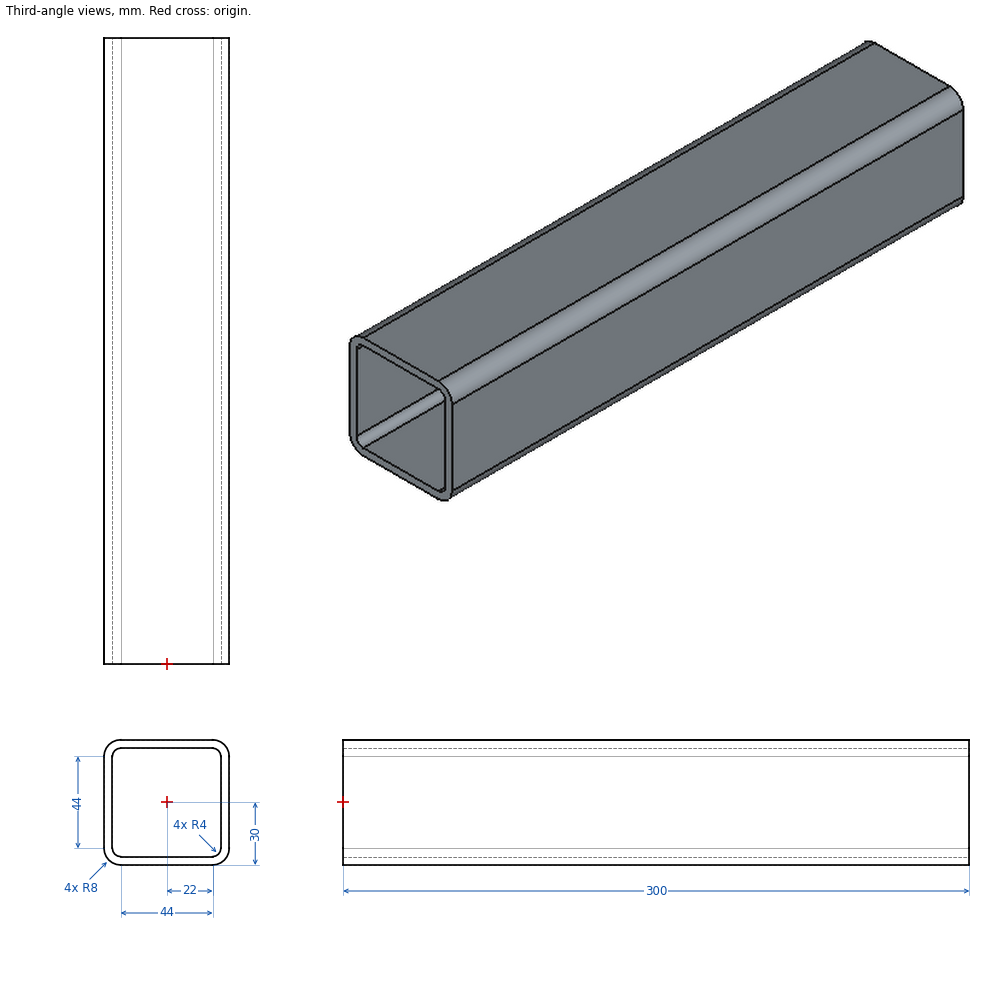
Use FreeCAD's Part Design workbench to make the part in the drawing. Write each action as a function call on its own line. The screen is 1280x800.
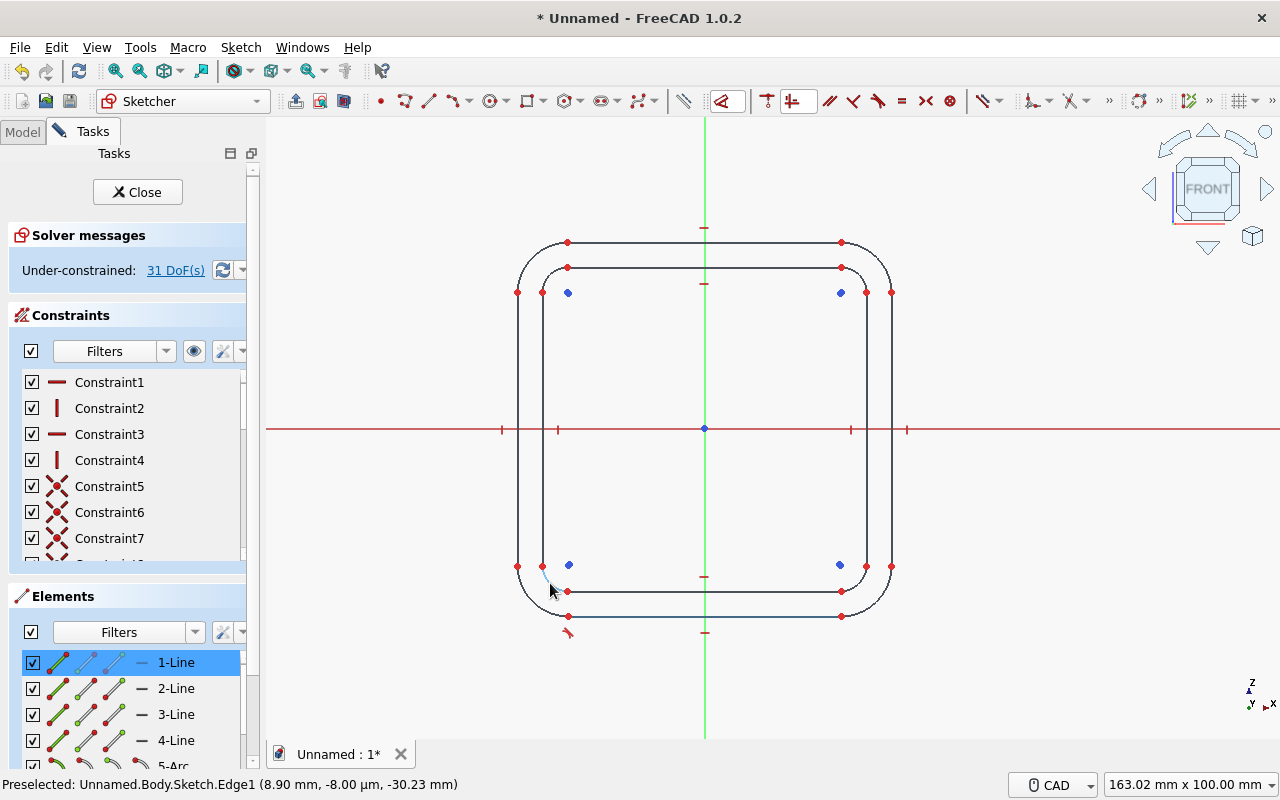
click(864, 611)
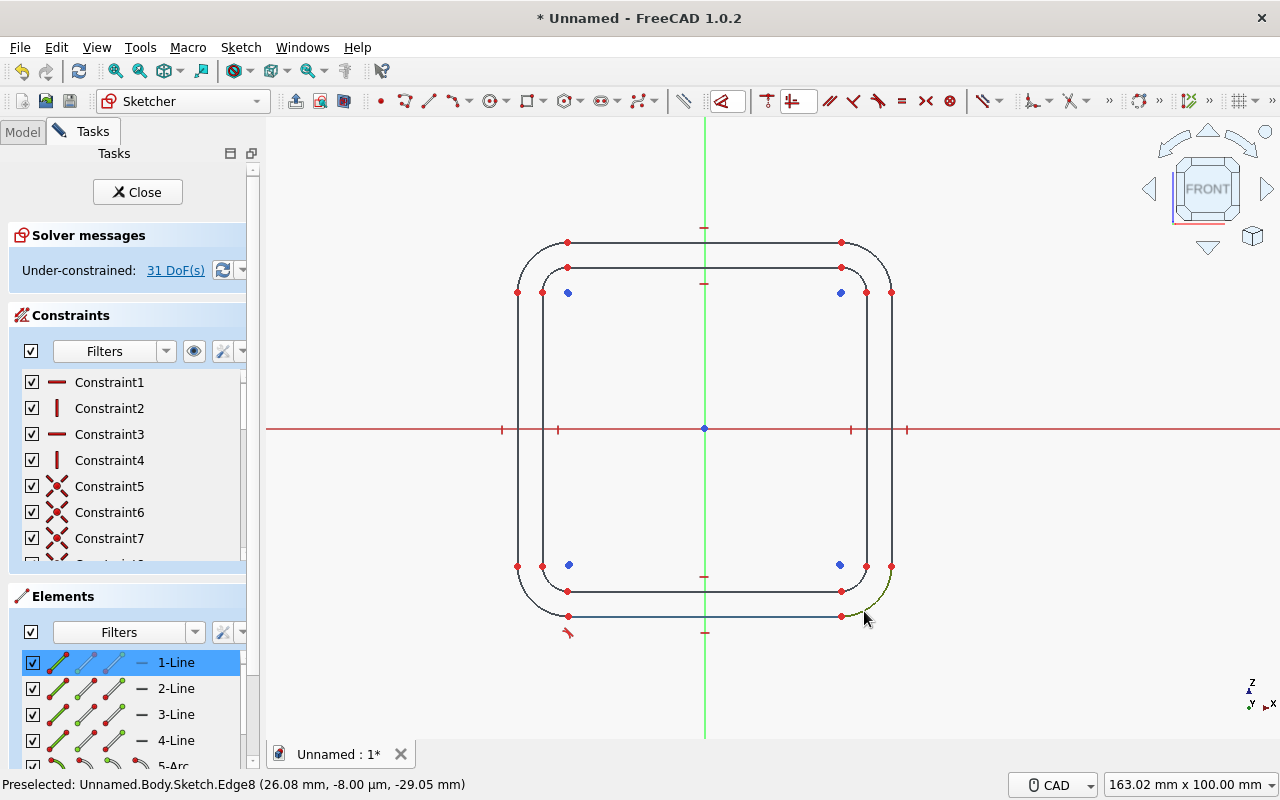
key(t)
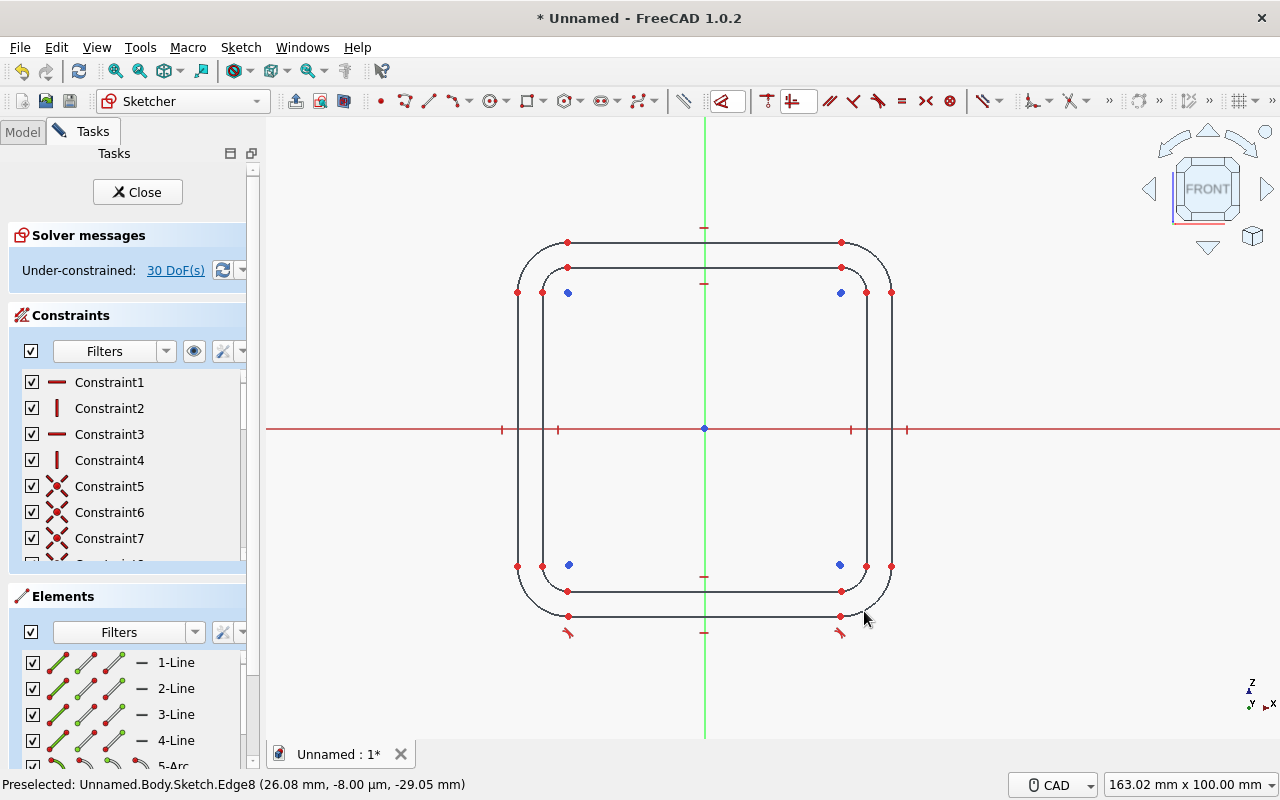
click(518, 484)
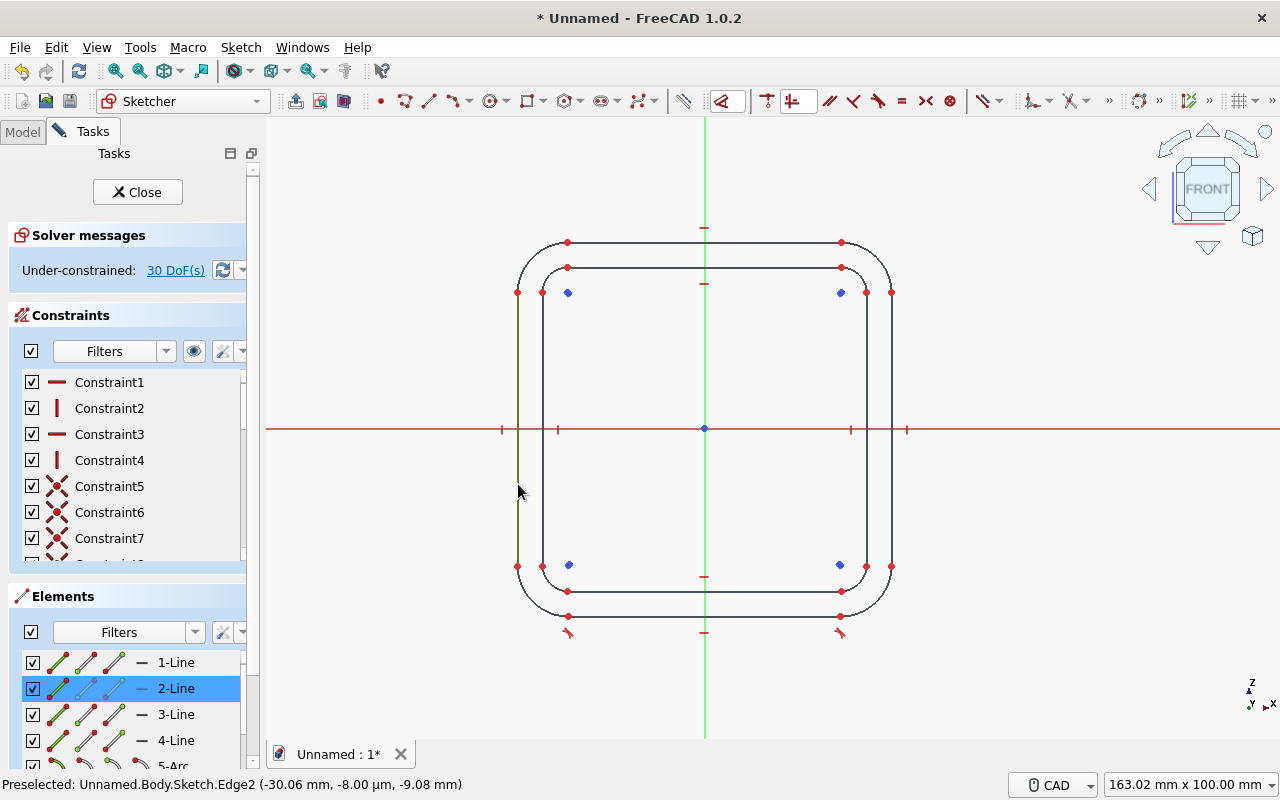
click(524, 589)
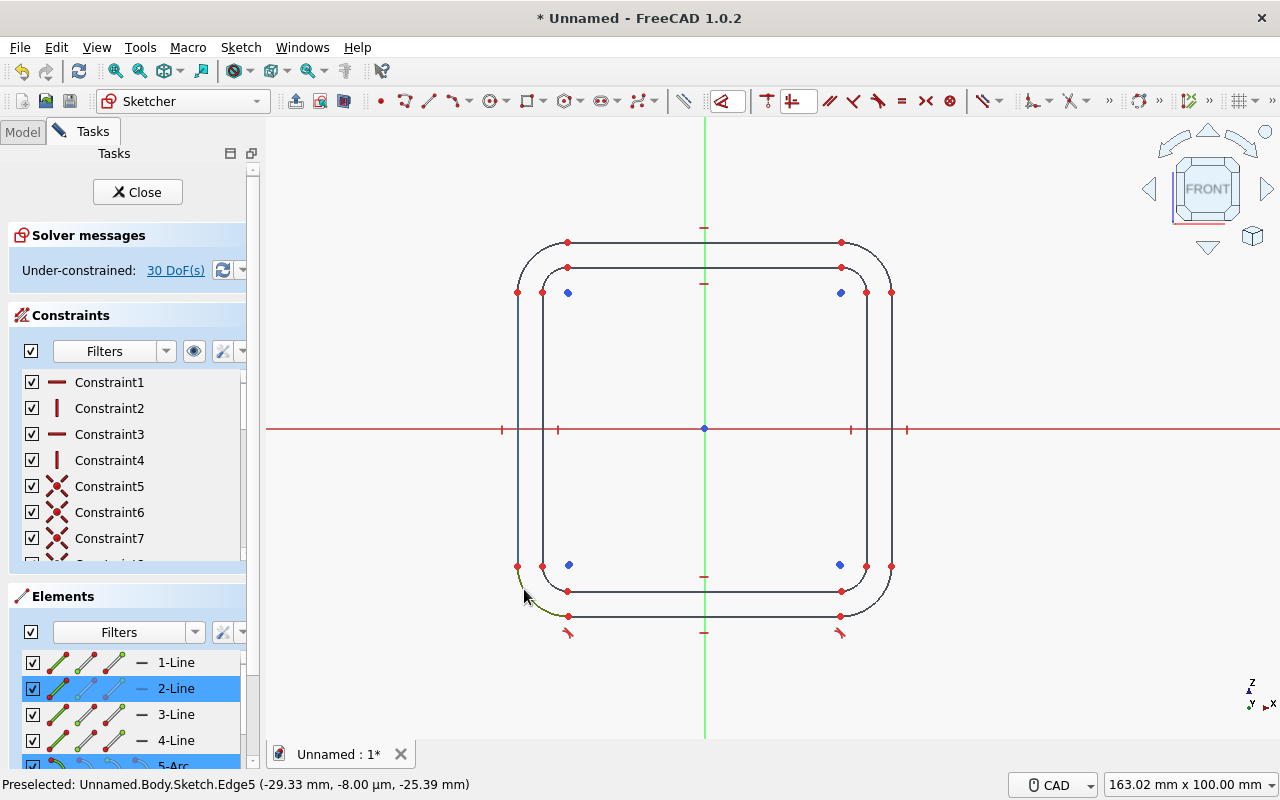
click(878, 102)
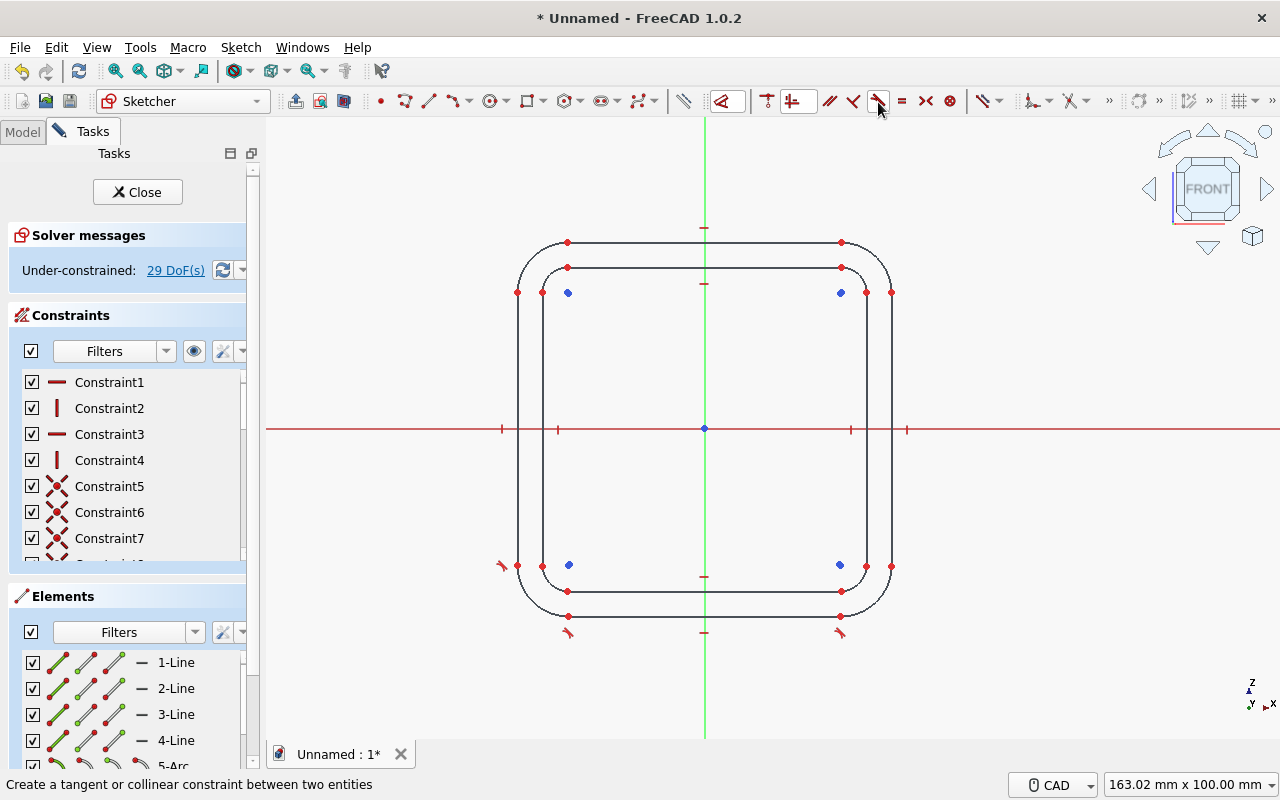
click(518, 483)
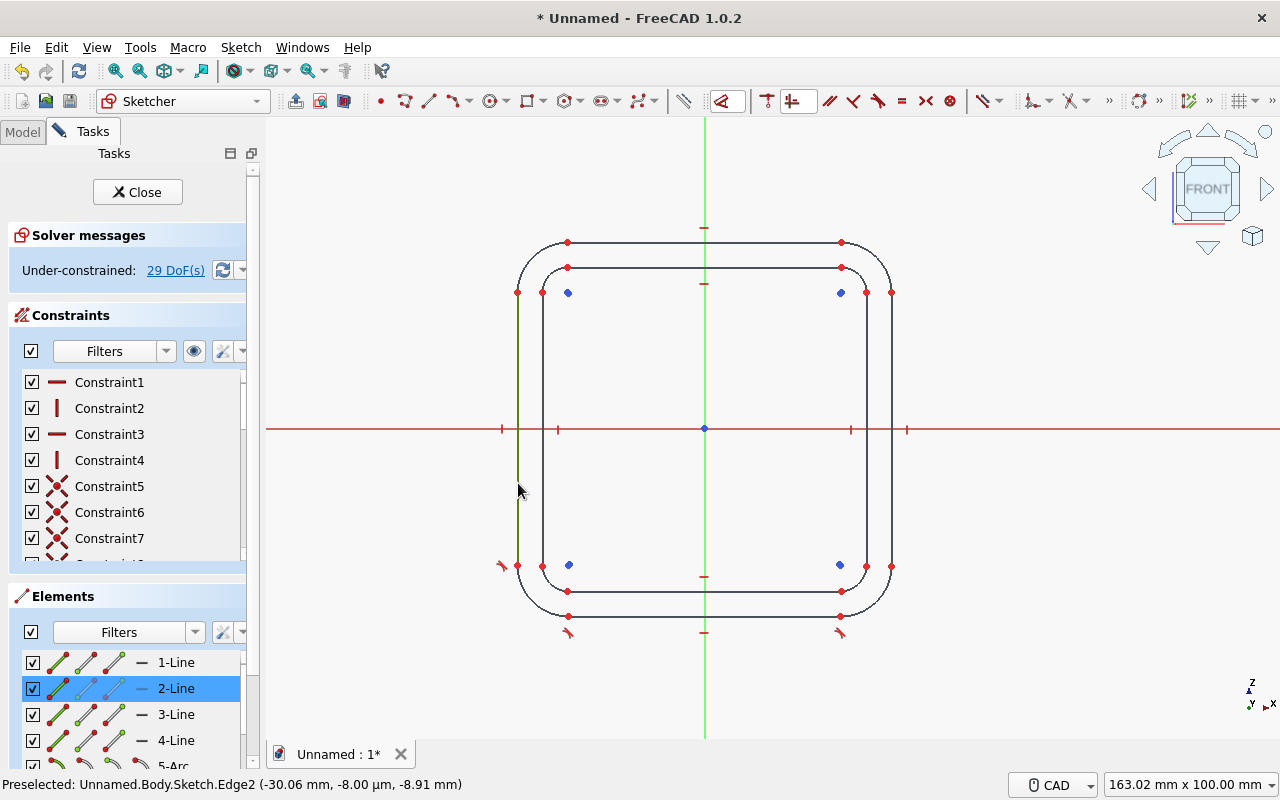
click(545, 248)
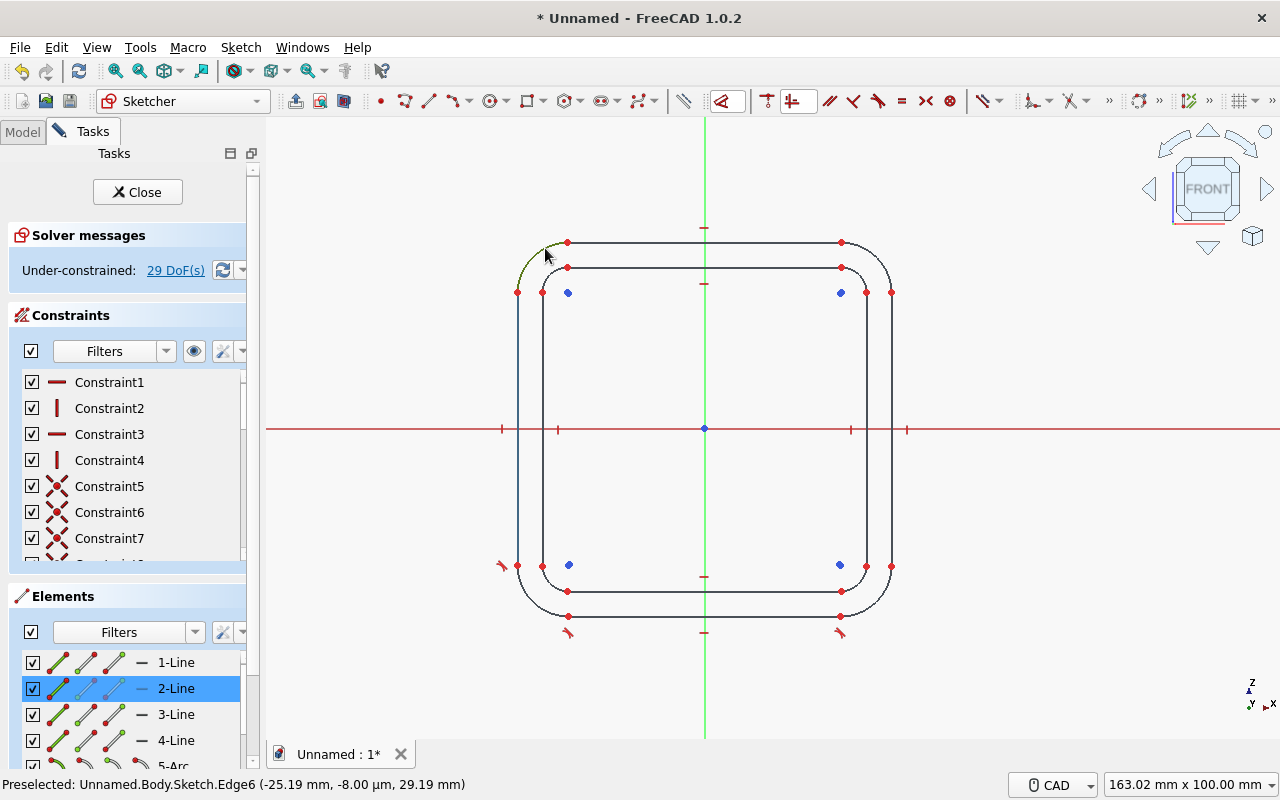
key(t)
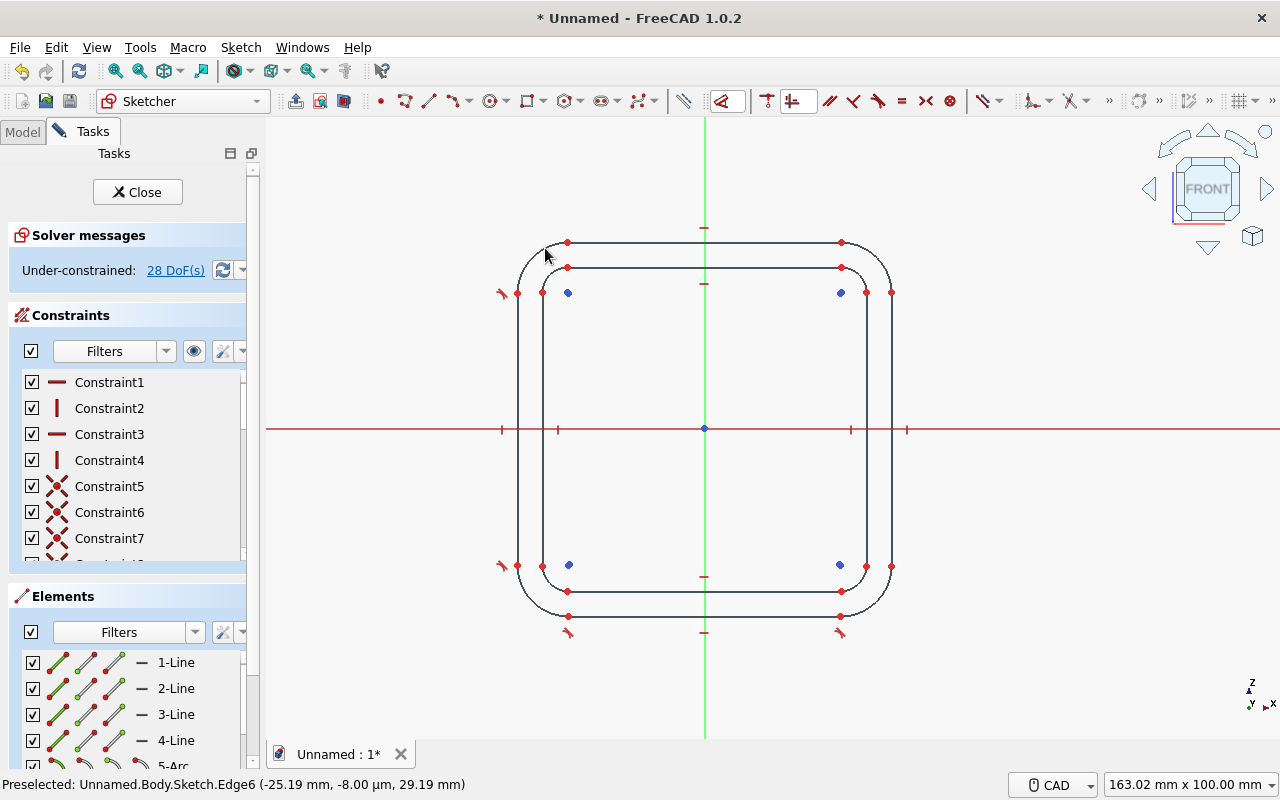
click(650, 243)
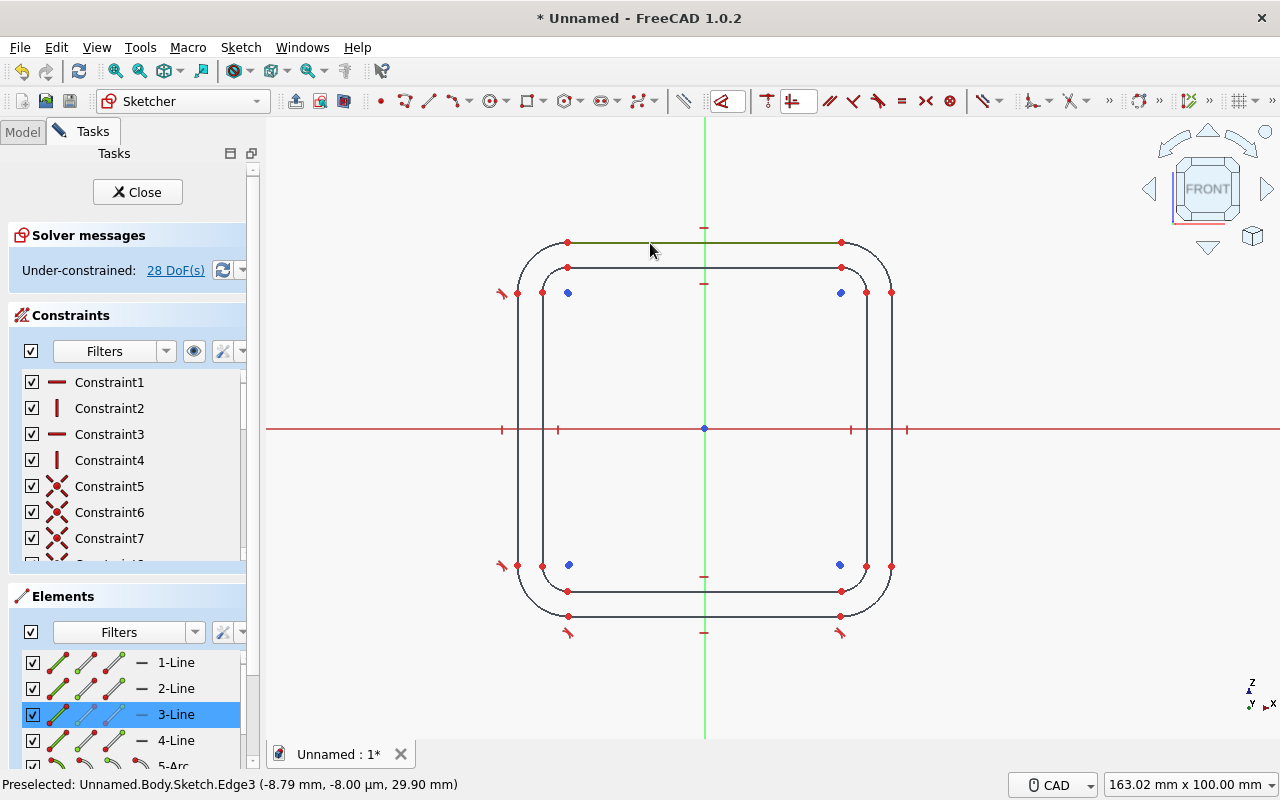
click(545, 249)